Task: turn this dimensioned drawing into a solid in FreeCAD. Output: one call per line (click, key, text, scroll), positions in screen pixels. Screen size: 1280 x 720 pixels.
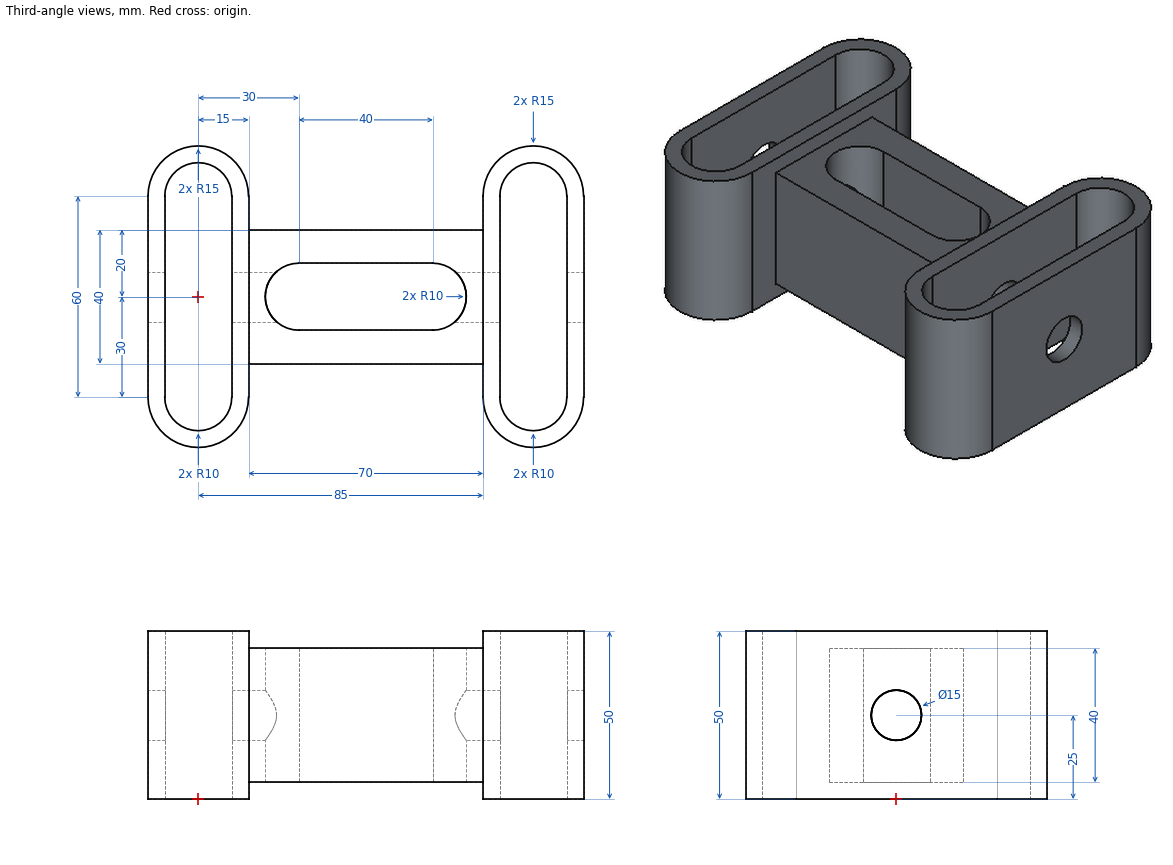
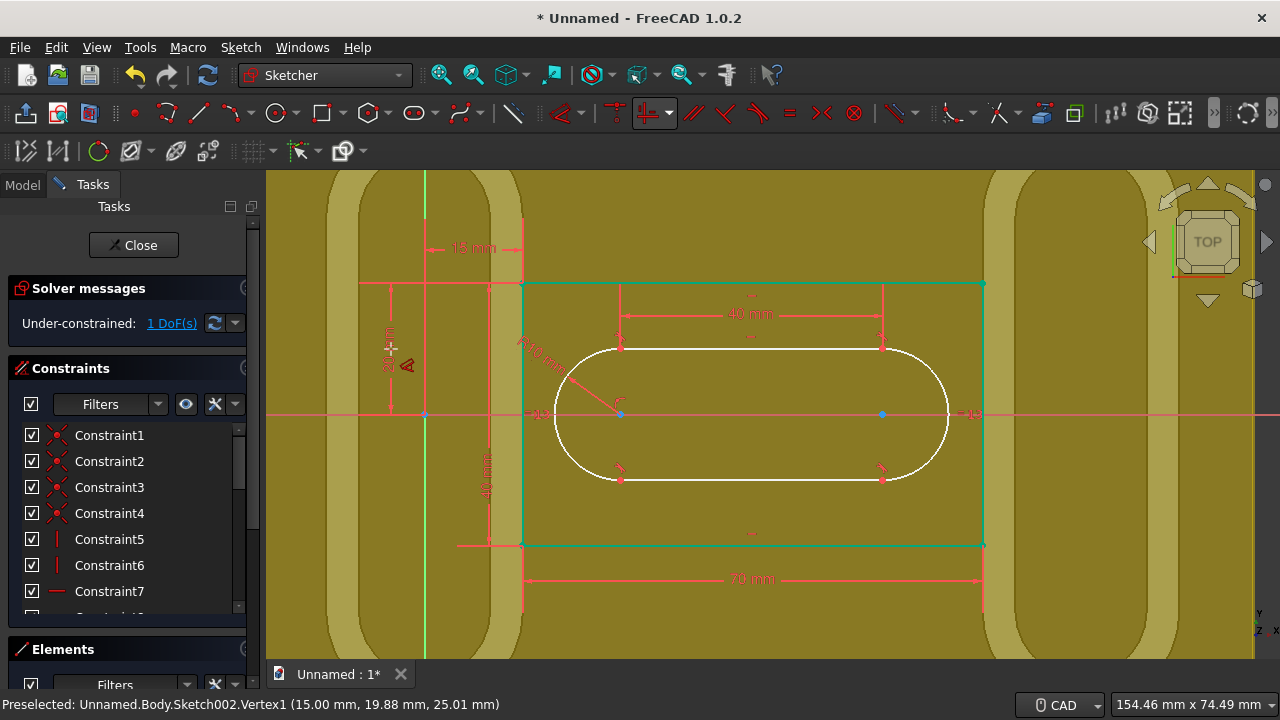
click(620, 349)
click(477, 315)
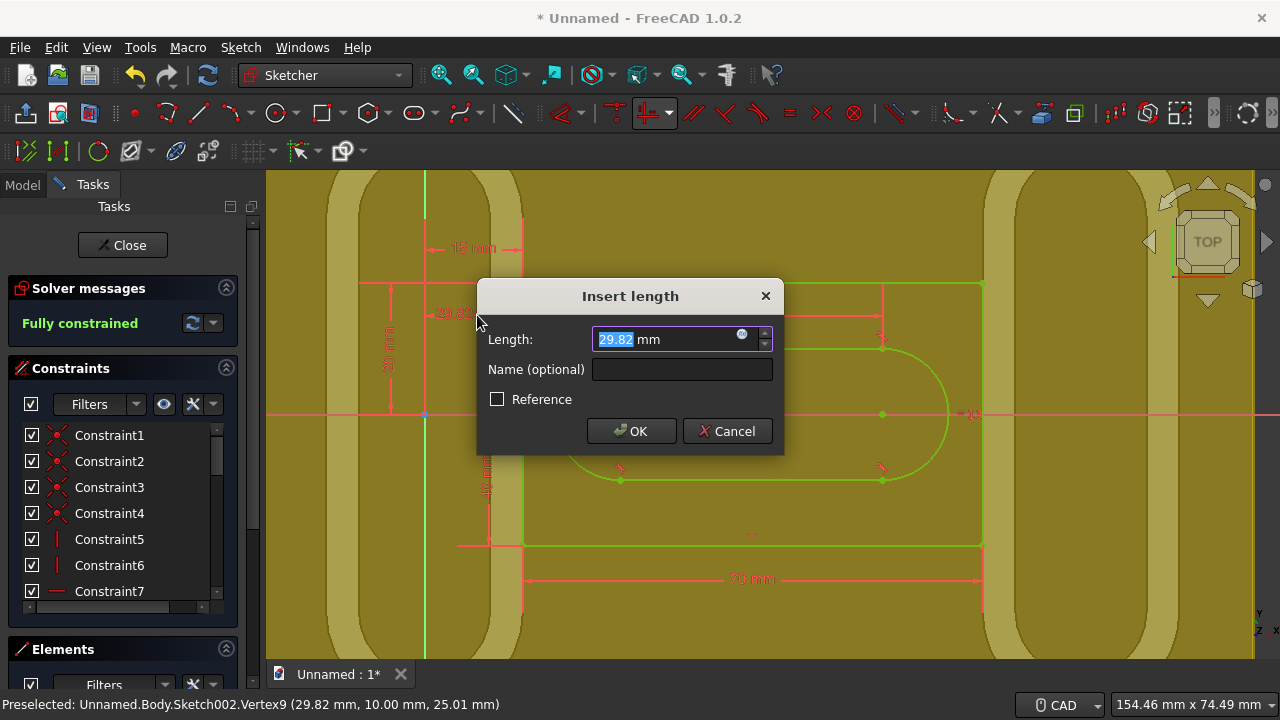
text(30)
key(Return)
key(Escape)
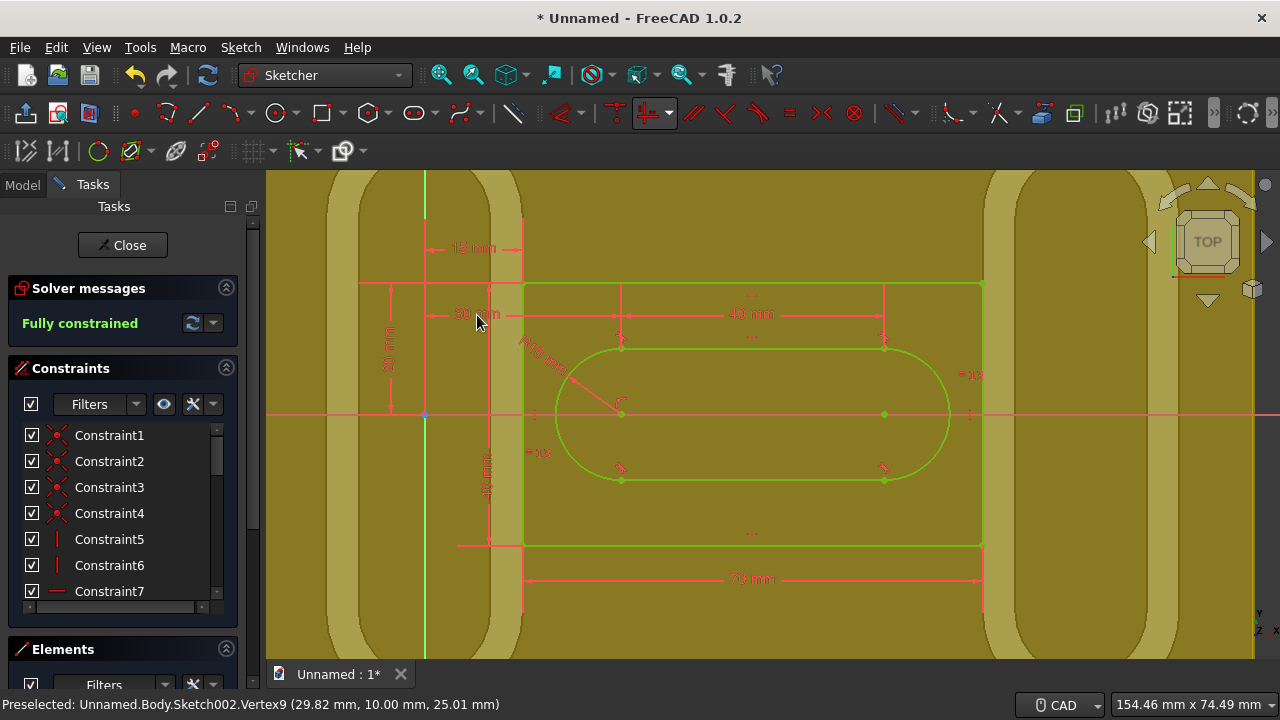
click(123, 245)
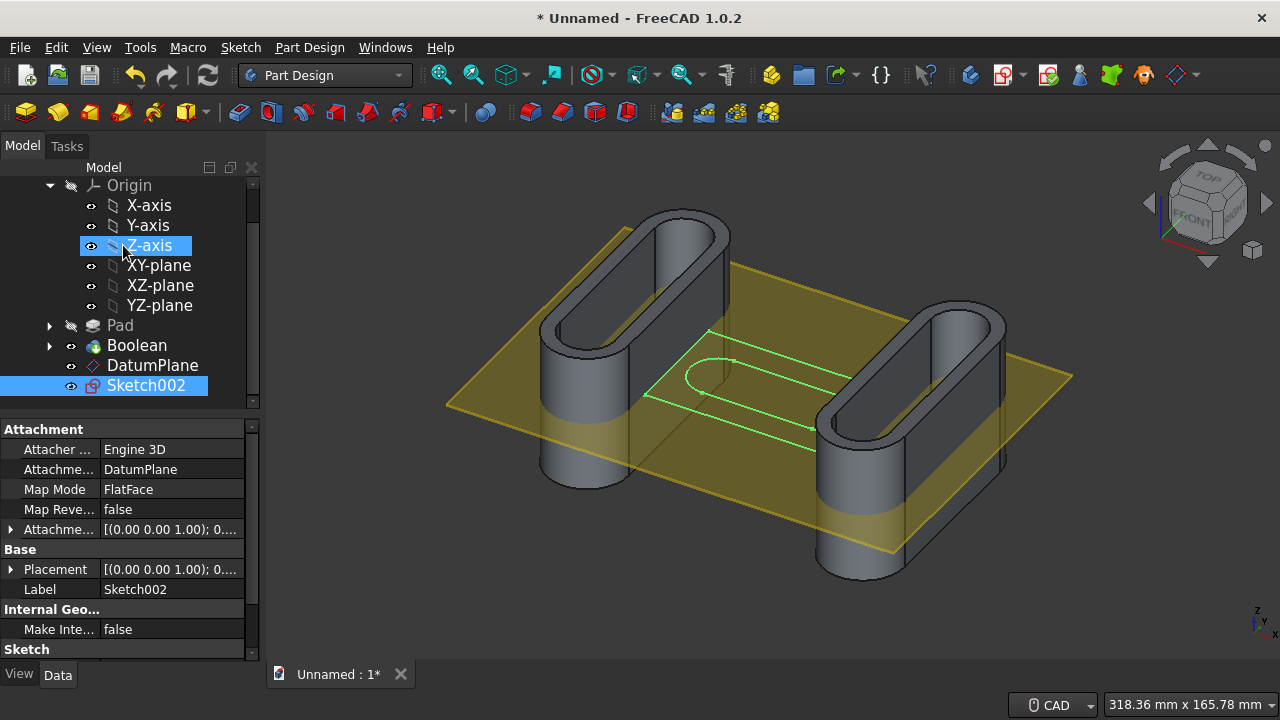
click(26, 112)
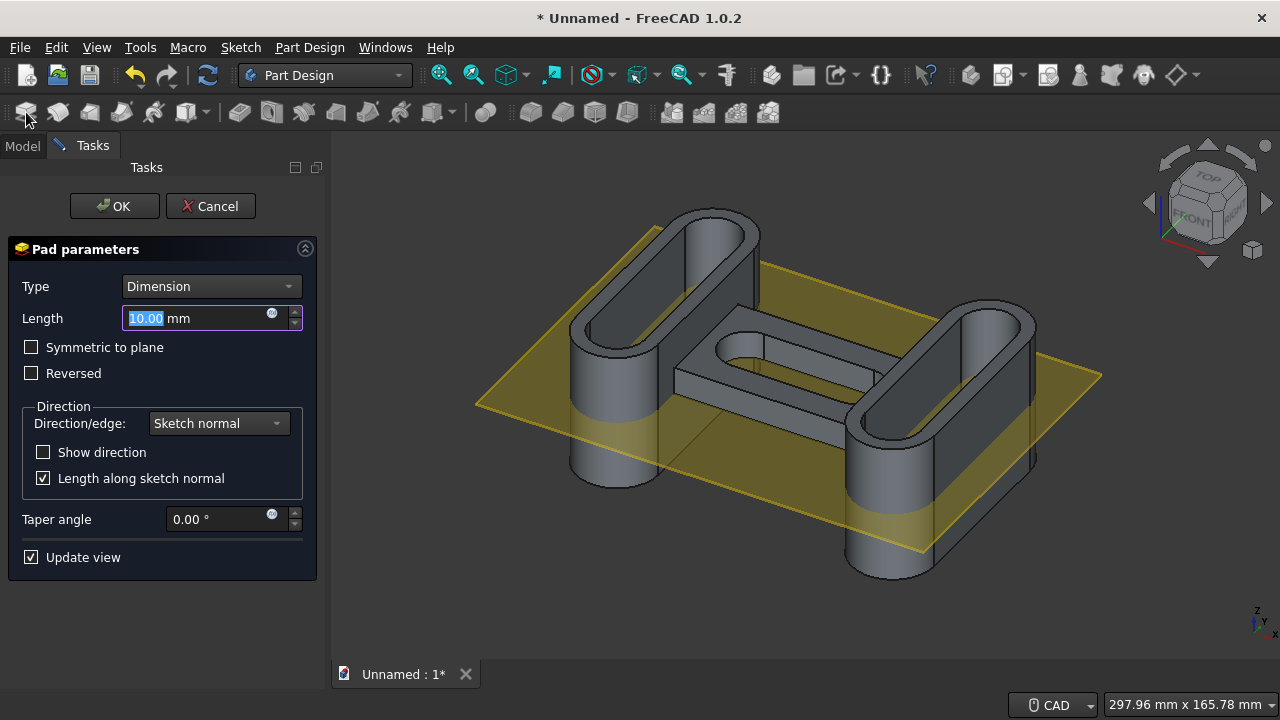
text(40)
key(Tab)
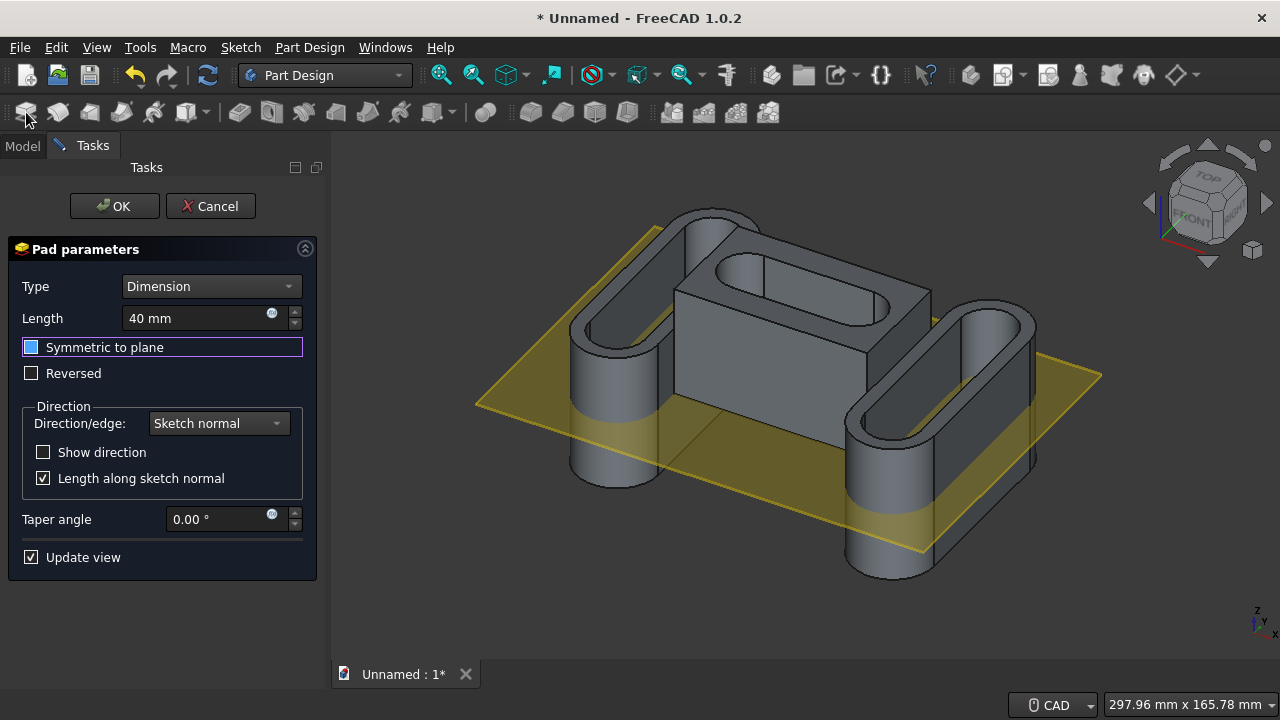
click(30, 347)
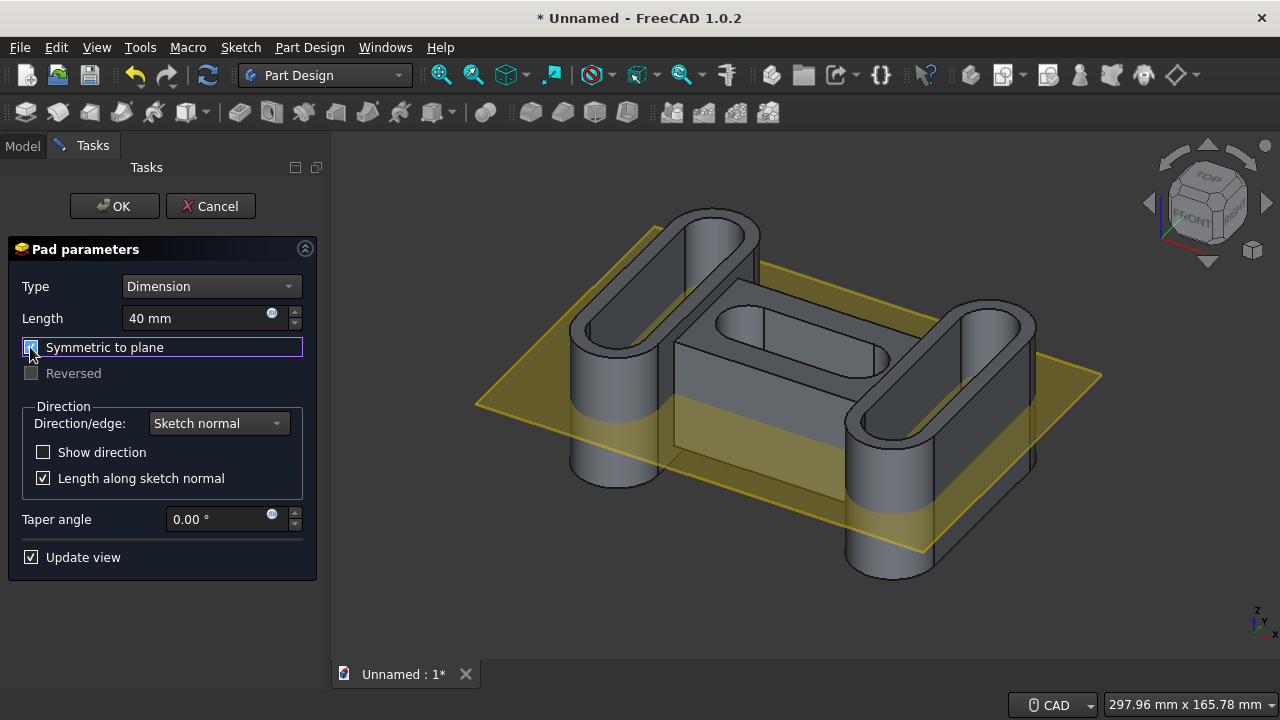
click(115, 206)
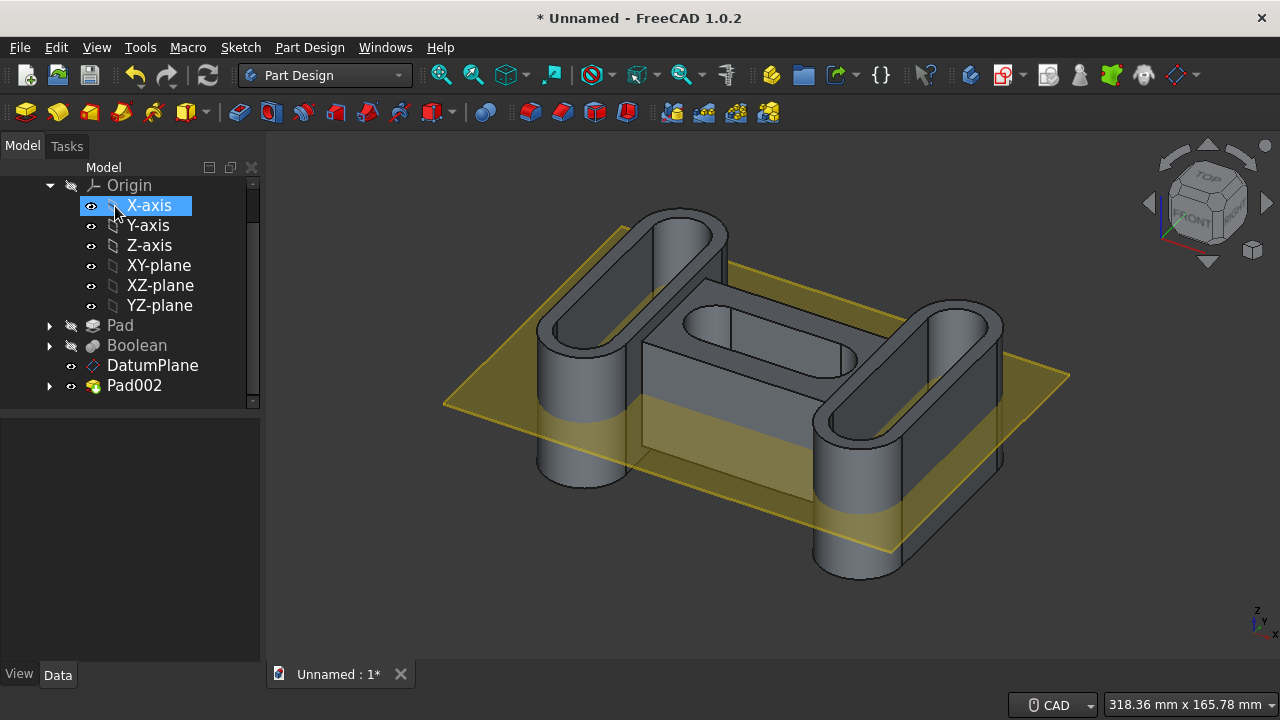
click(116, 366)
key(space)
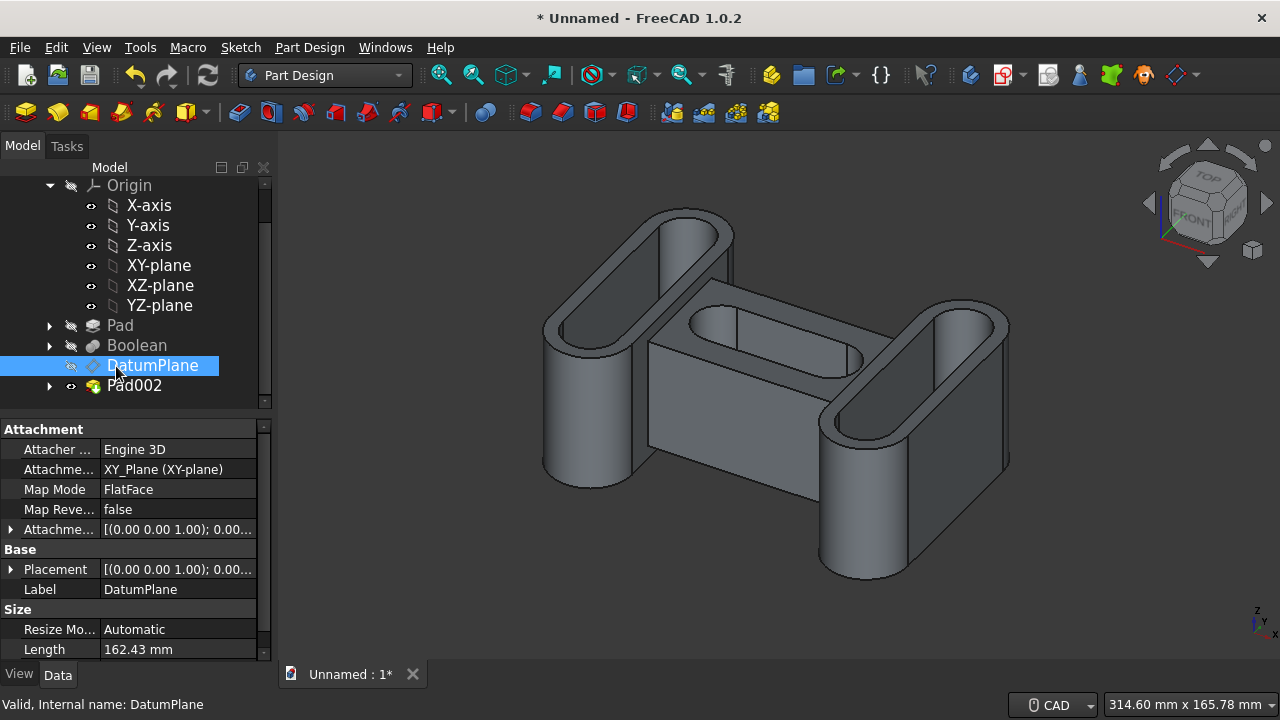
key(6)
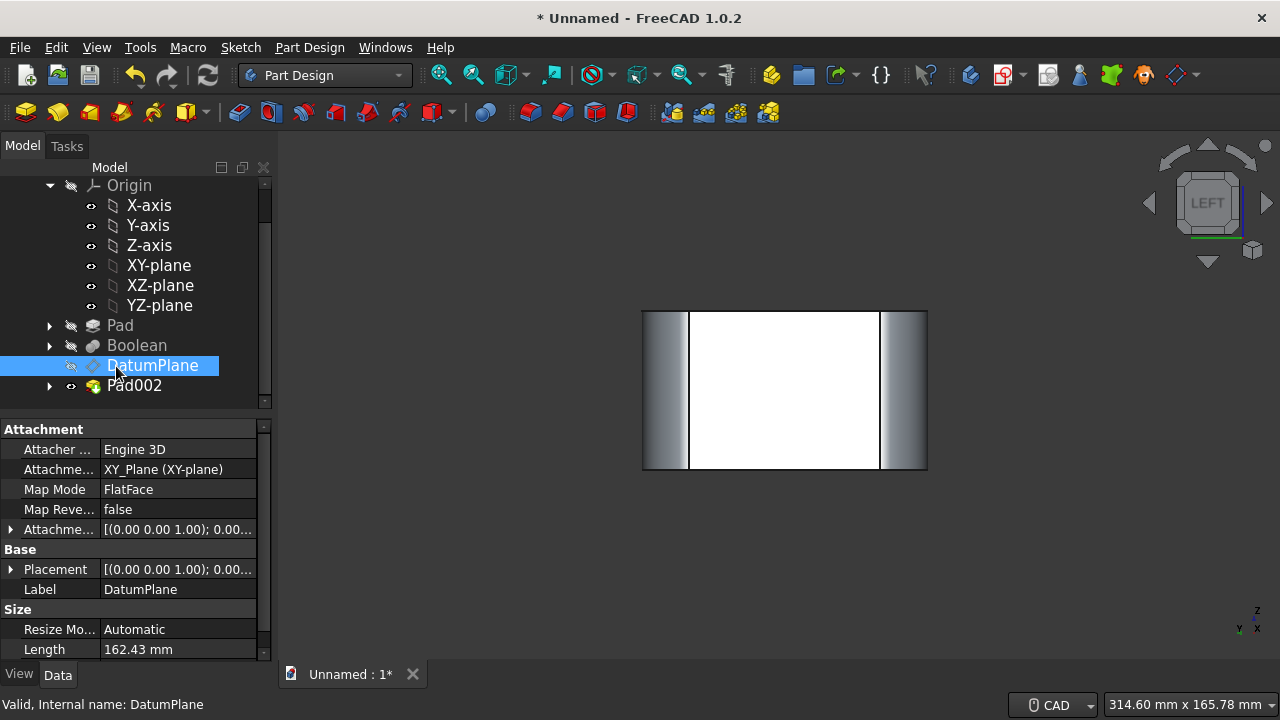
click(442, 76)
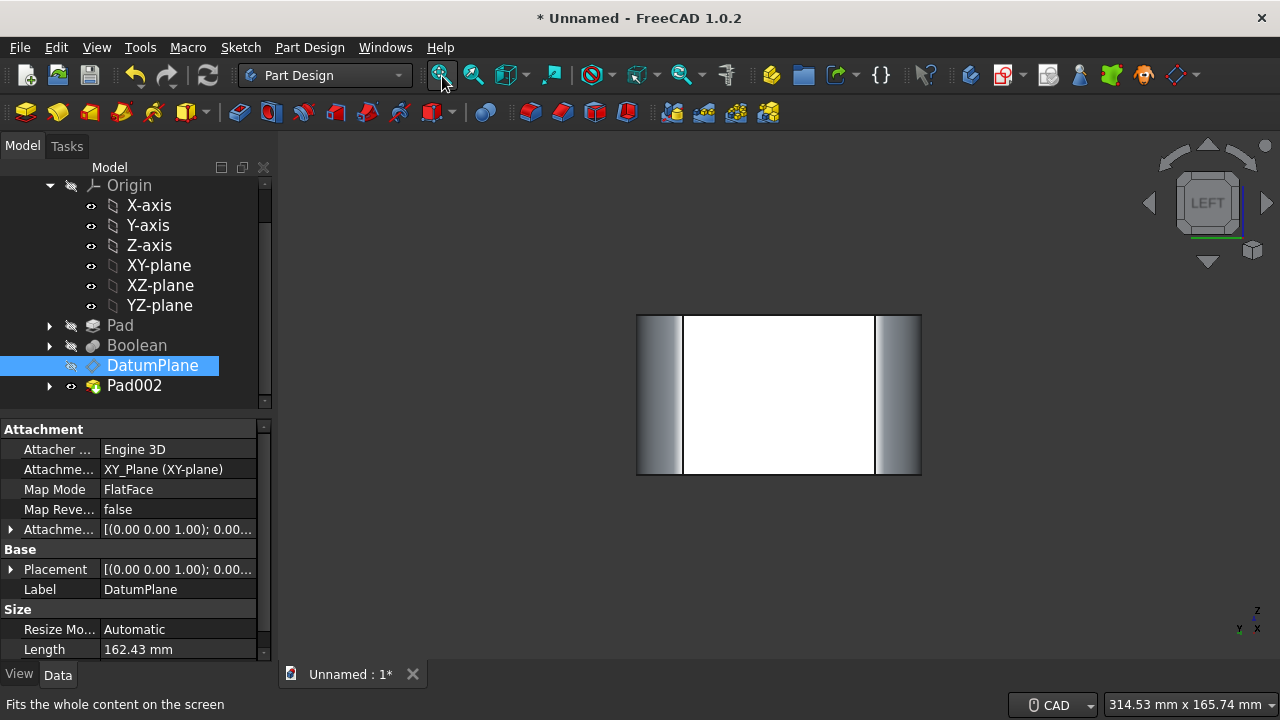
click(779, 394)